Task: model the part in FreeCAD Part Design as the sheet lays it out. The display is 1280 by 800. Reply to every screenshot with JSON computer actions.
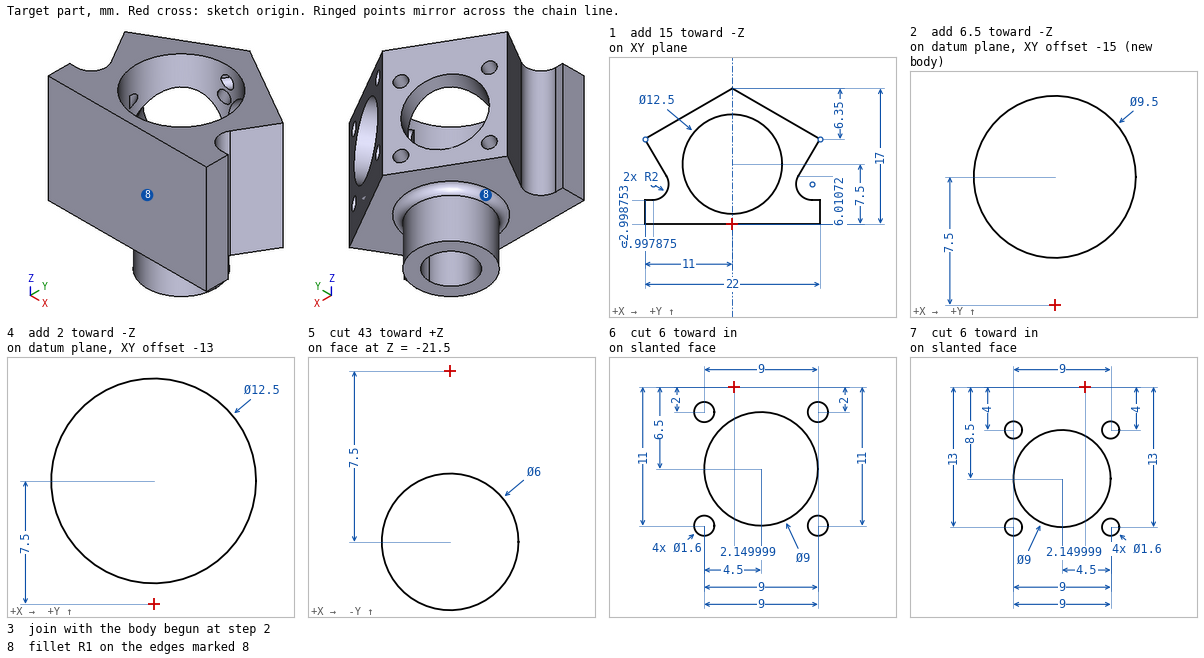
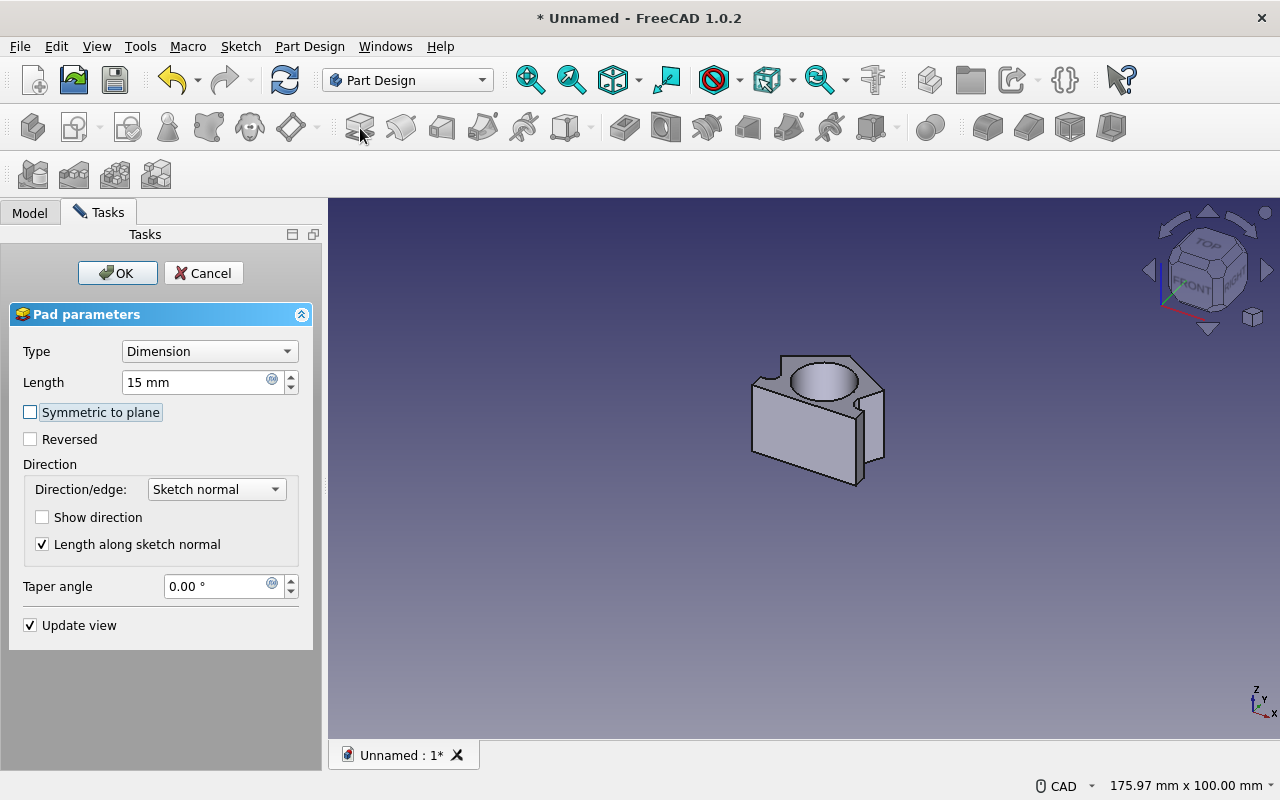
{"action": "left_click", "coordinate": [31, 439]}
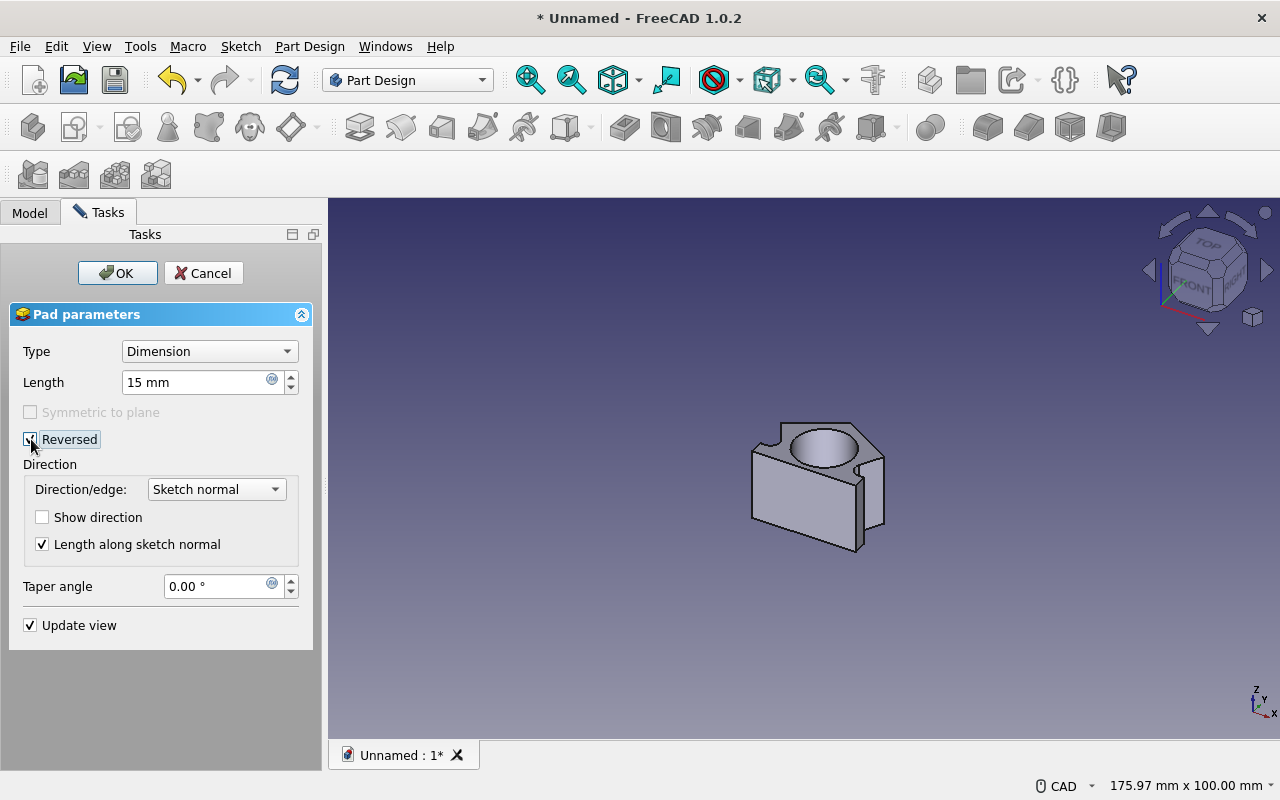
{"action": "left_click", "coordinate": [118, 273]}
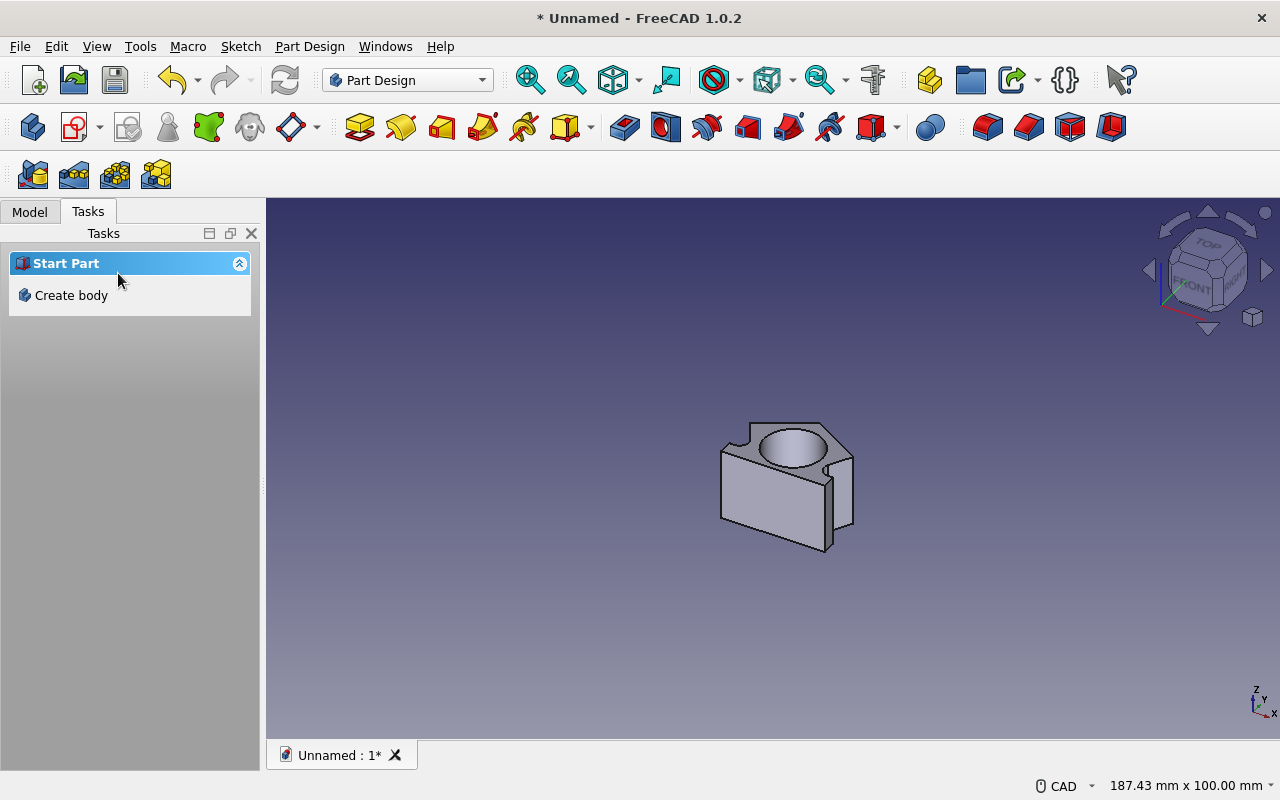
{"action": "left_click", "coordinate": [531, 80]}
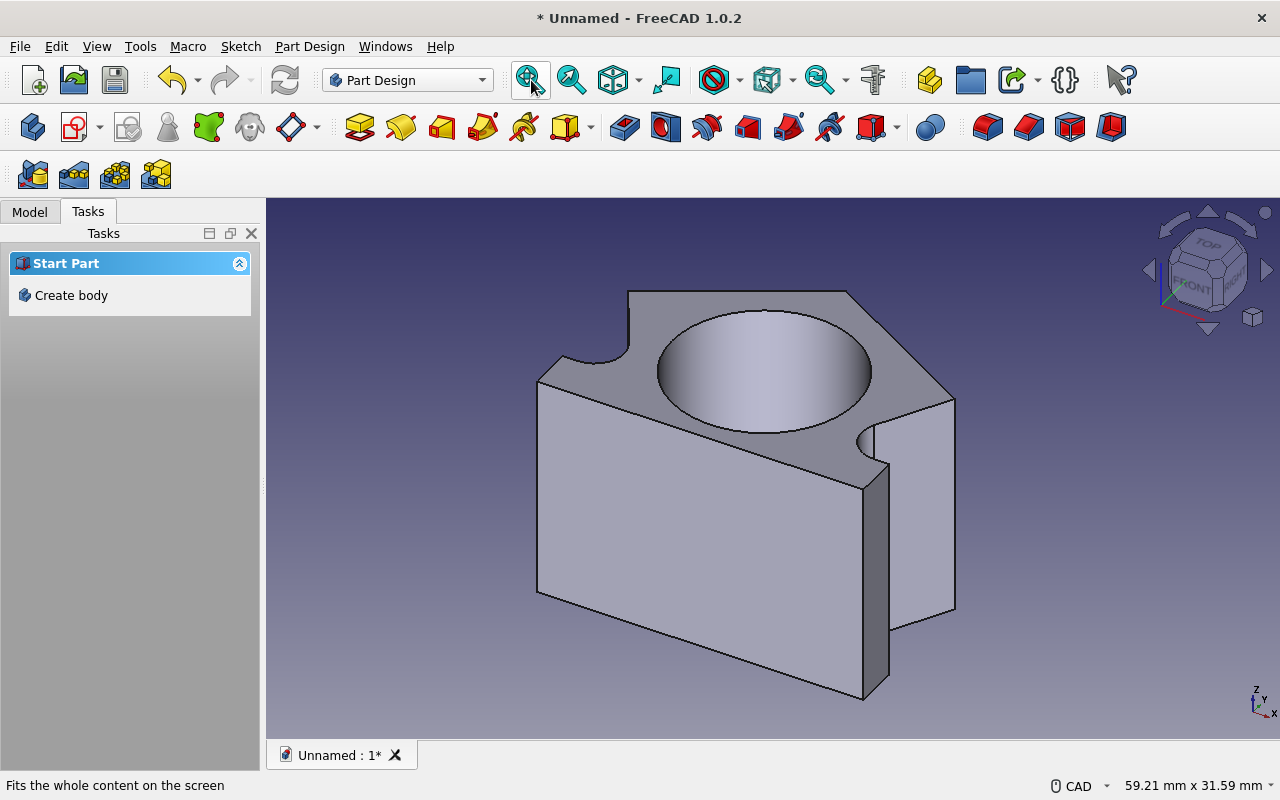
{"action": "left_click", "coordinate": [33, 128]}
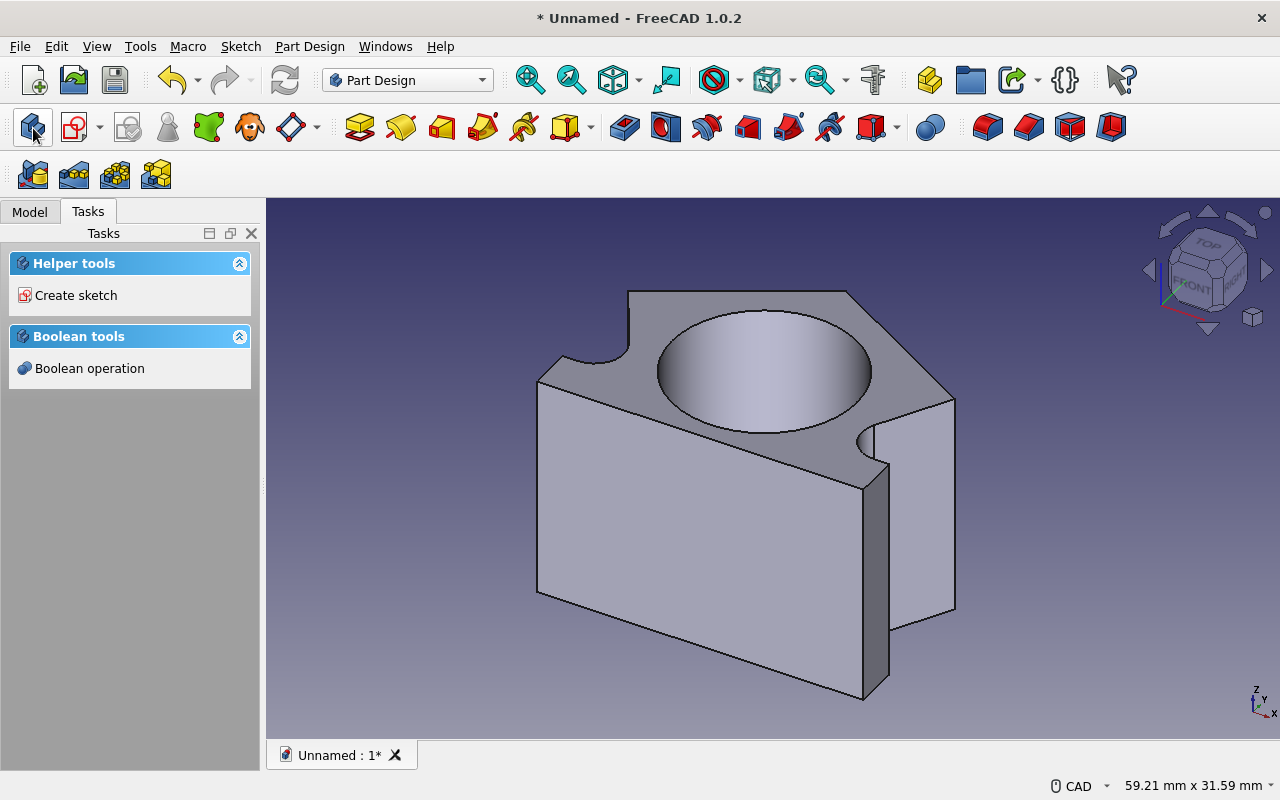
{"action": "left_click", "coordinate": [30, 212]}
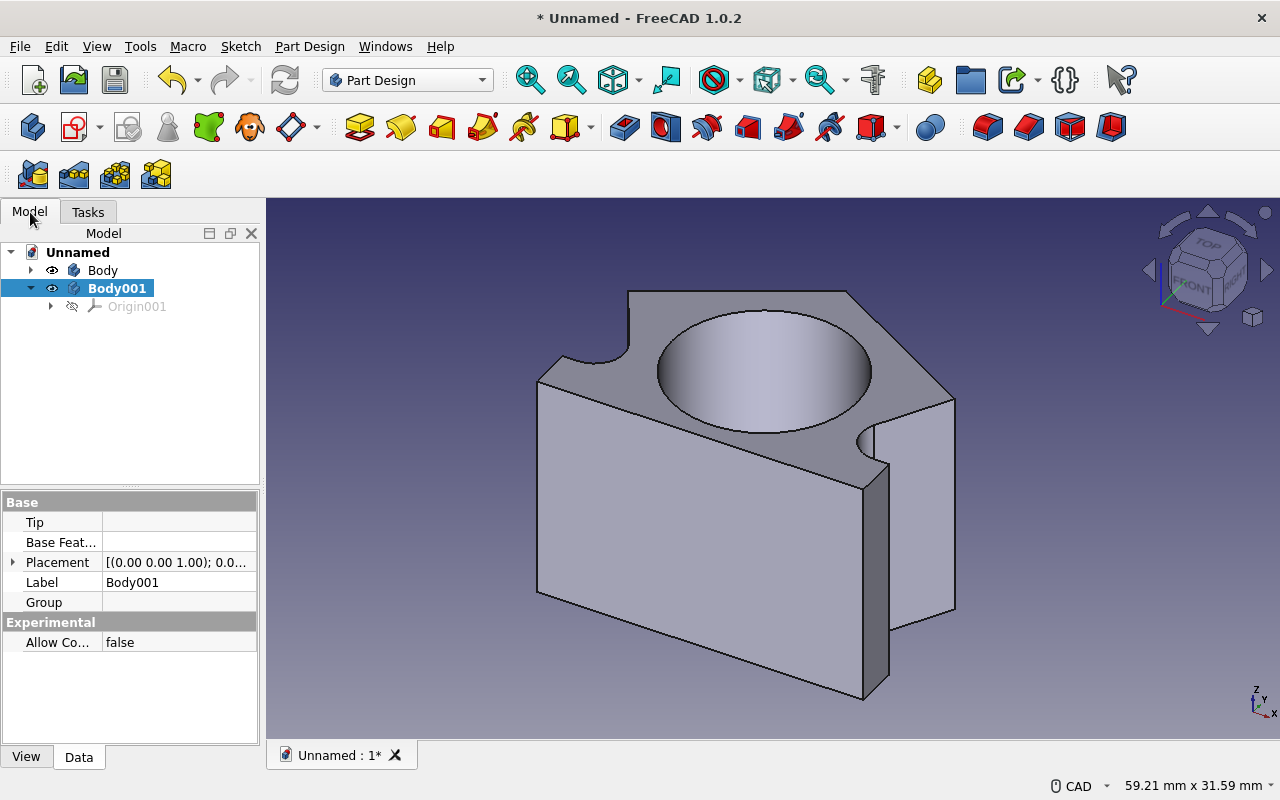
{"action": "left_click", "coordinate": [51, 306]}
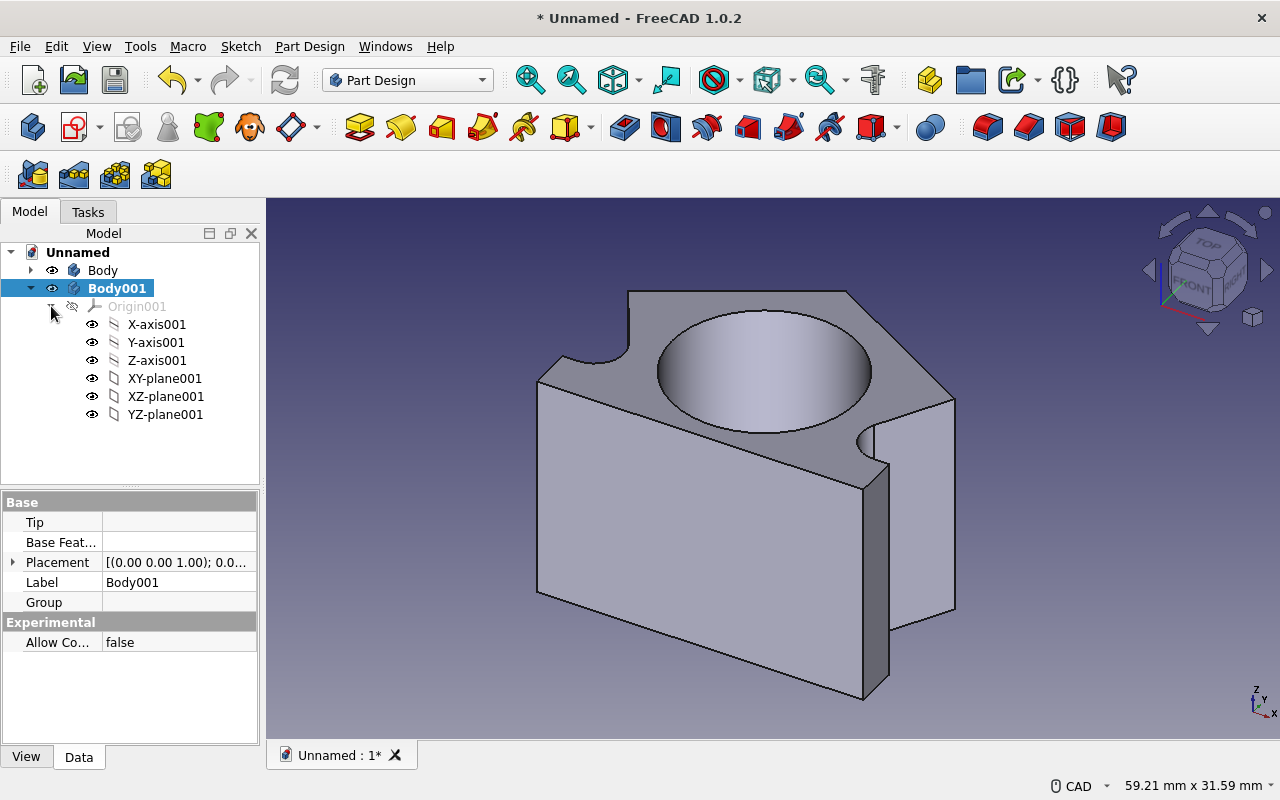
{"action": "left_click", "coordinate": [137, 378]}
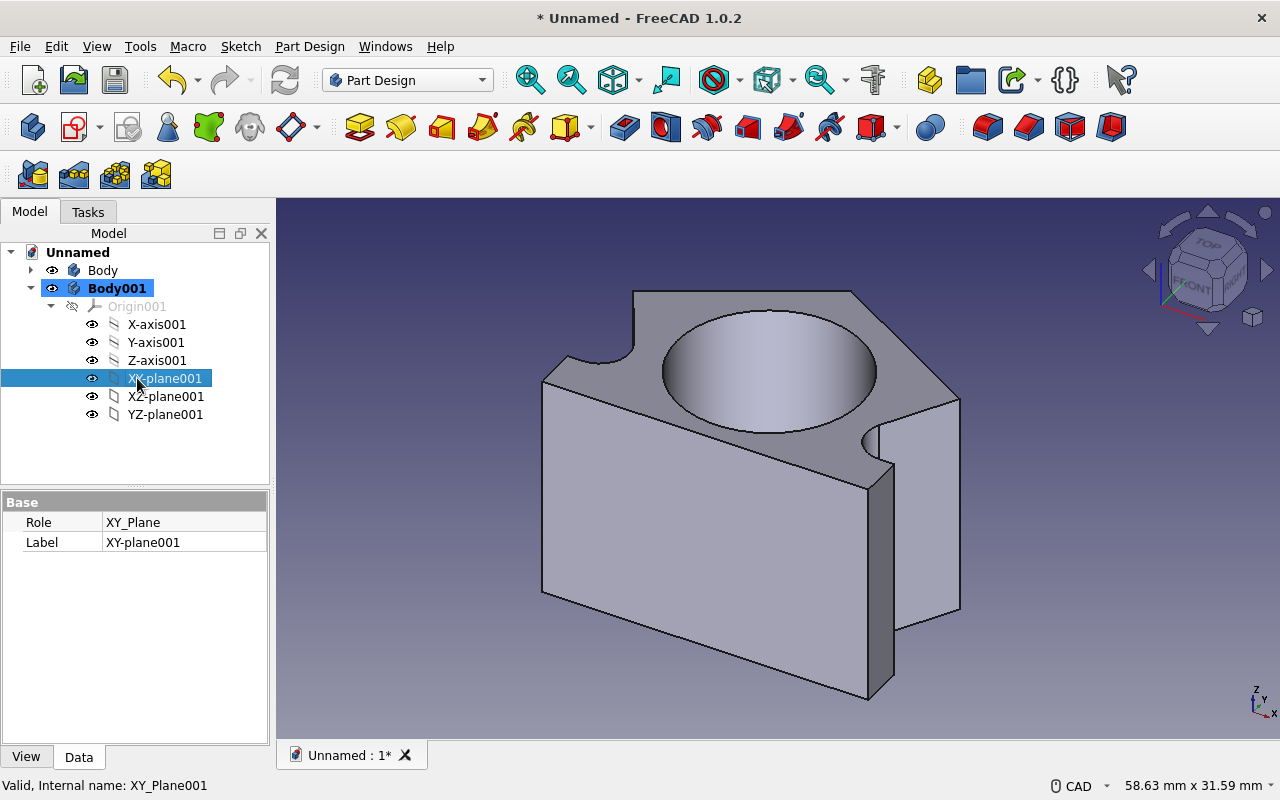
{"action": "left_click", "coordinate": [290, 128]}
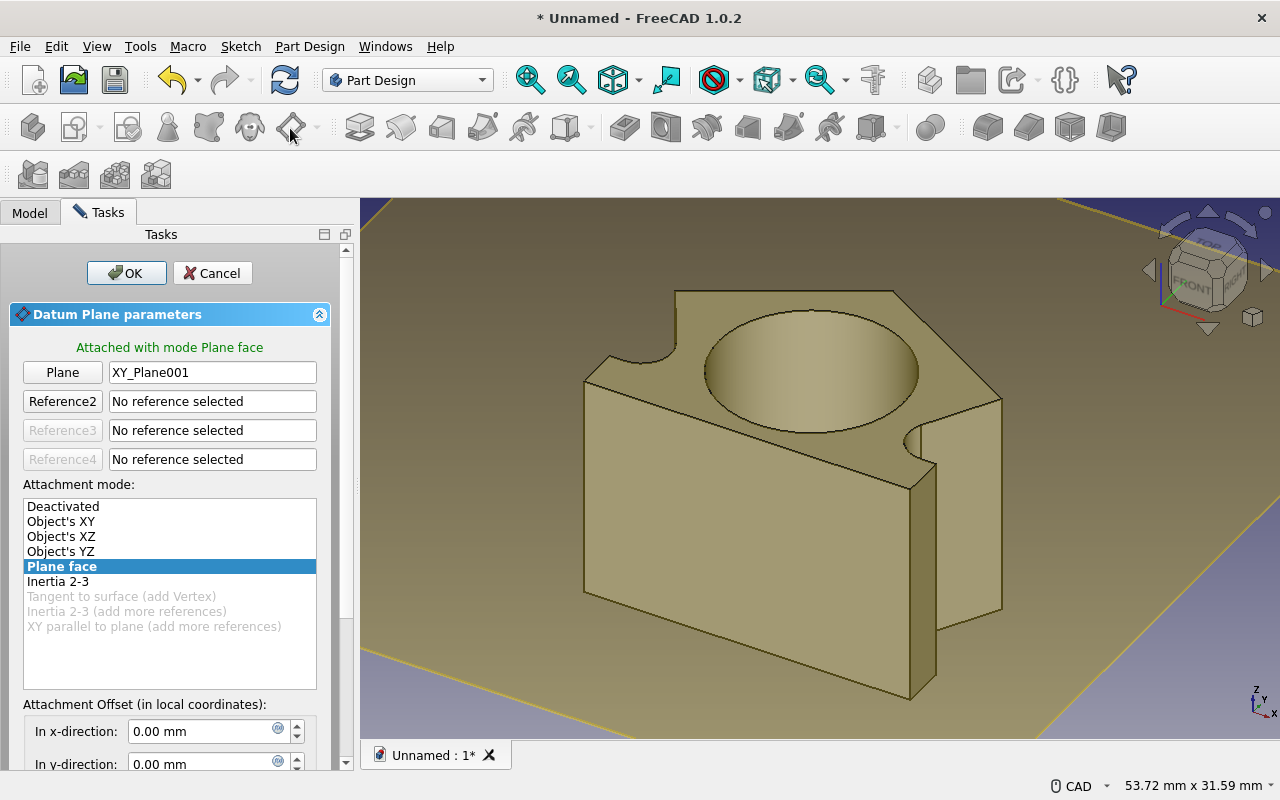
{"action": "scroll", "coordinate": [346, 507], "scroll_direction": "down", "scroll_amount": 2}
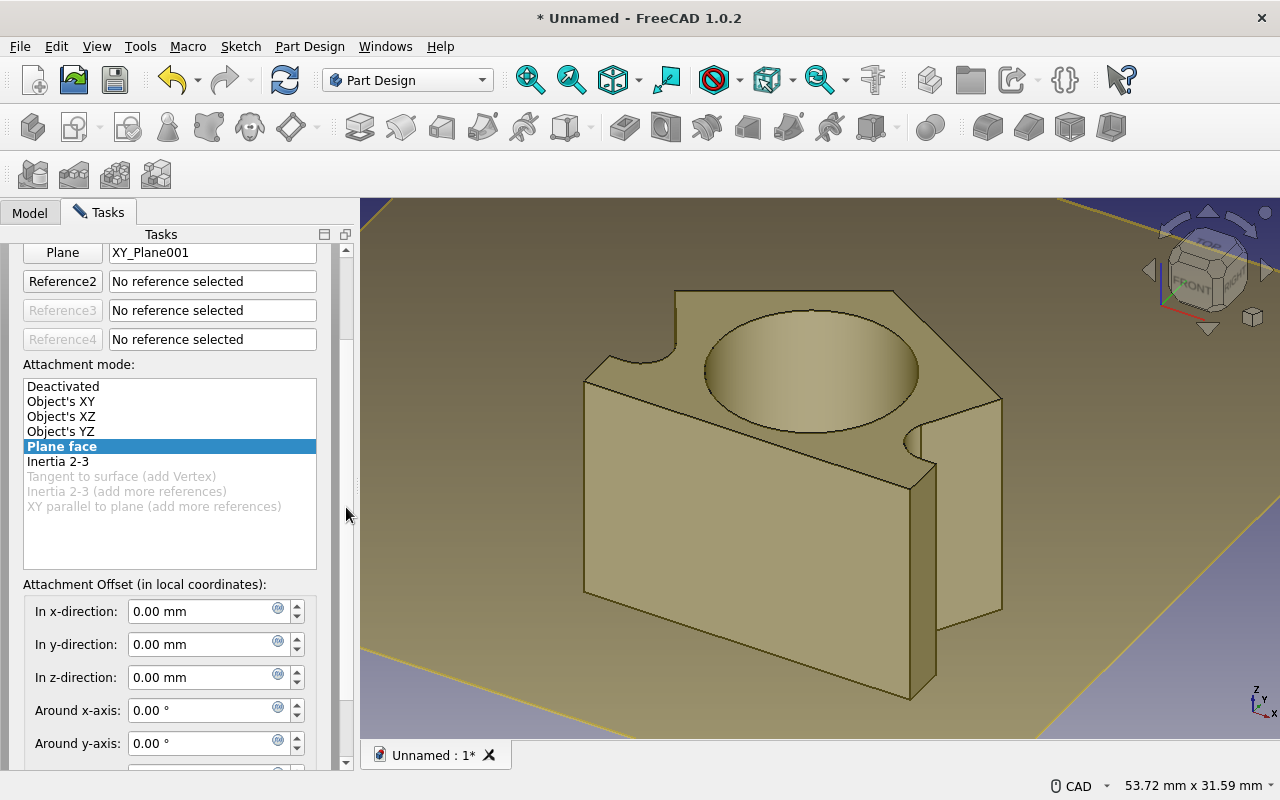
{"action": "triple_click", "coordinate": [210, 678]}